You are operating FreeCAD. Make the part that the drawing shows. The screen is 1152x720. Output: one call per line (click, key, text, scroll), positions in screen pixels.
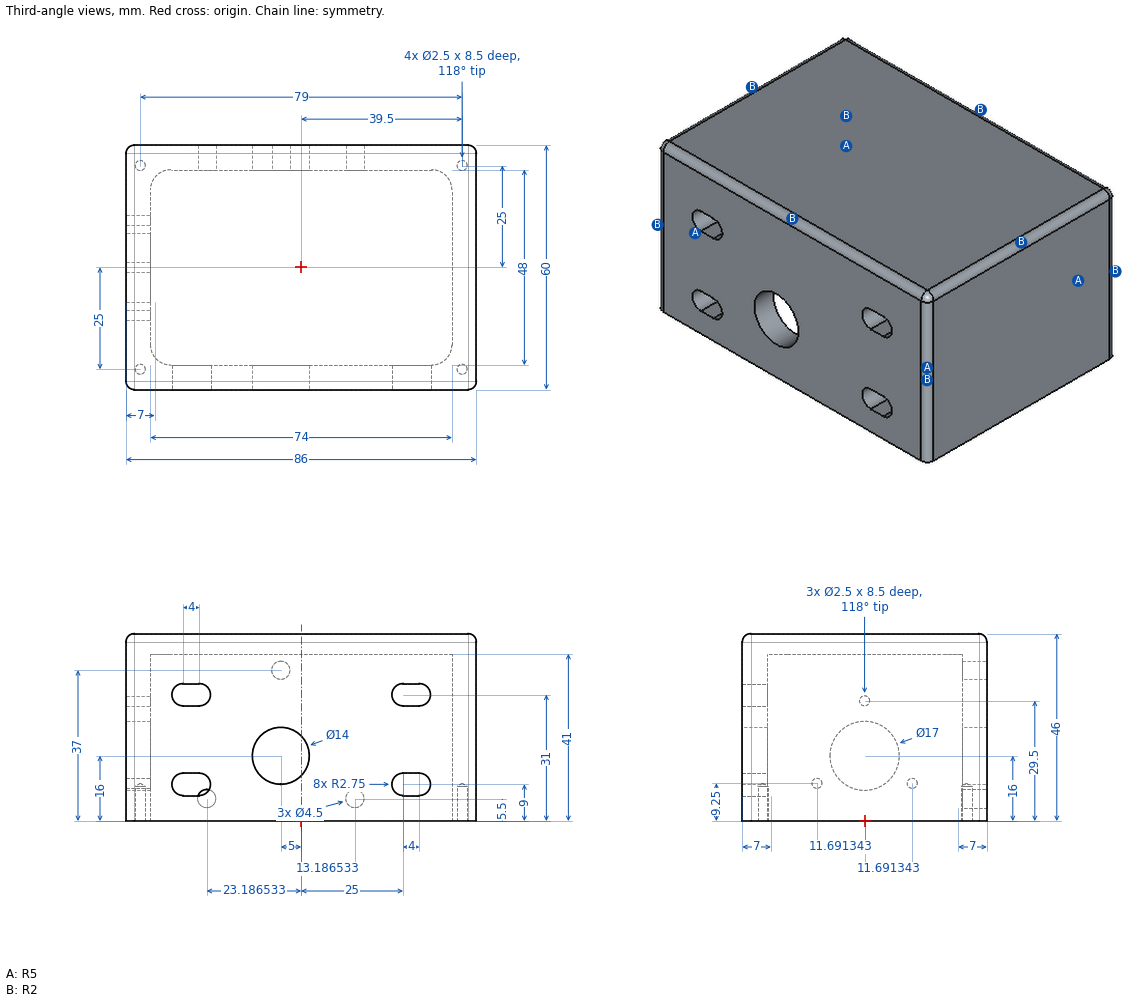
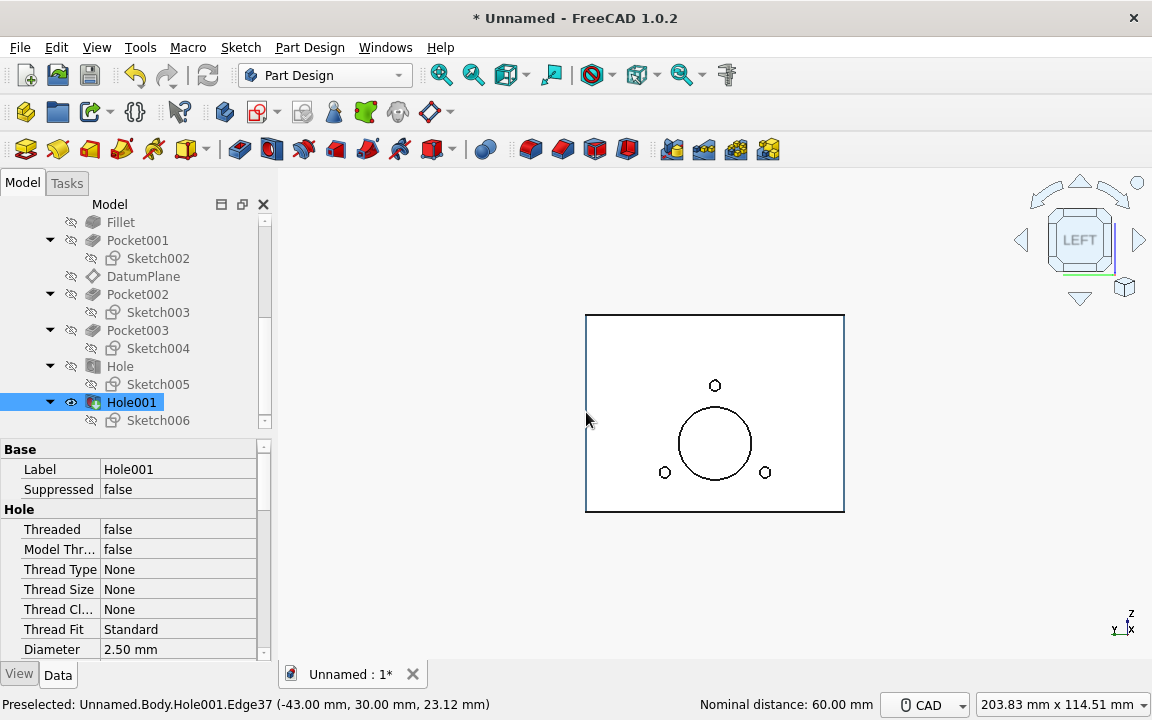
key(0)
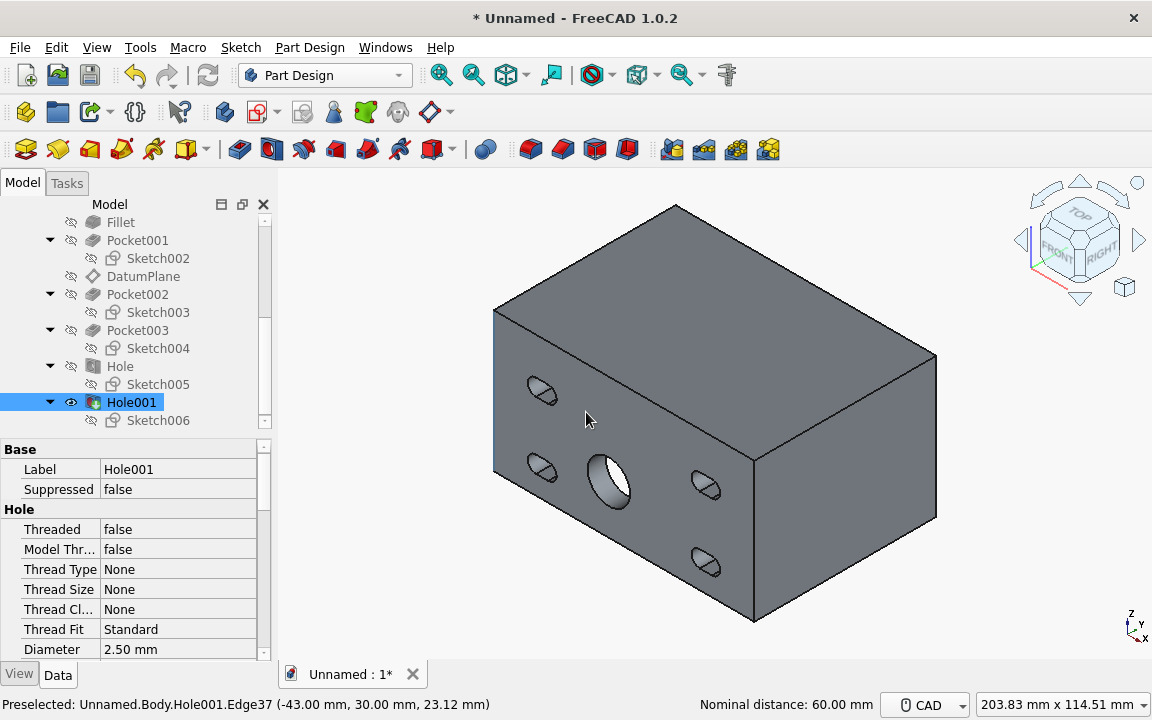
click(752, 353, ctrl)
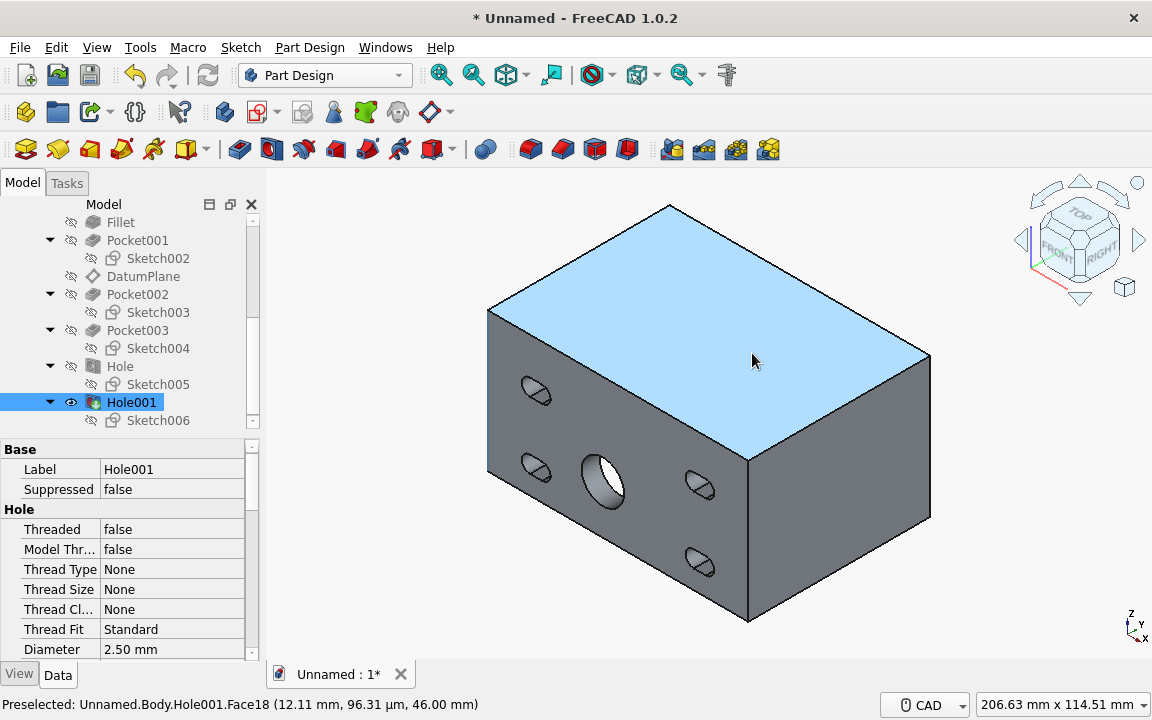
click(748, 540, ctrl)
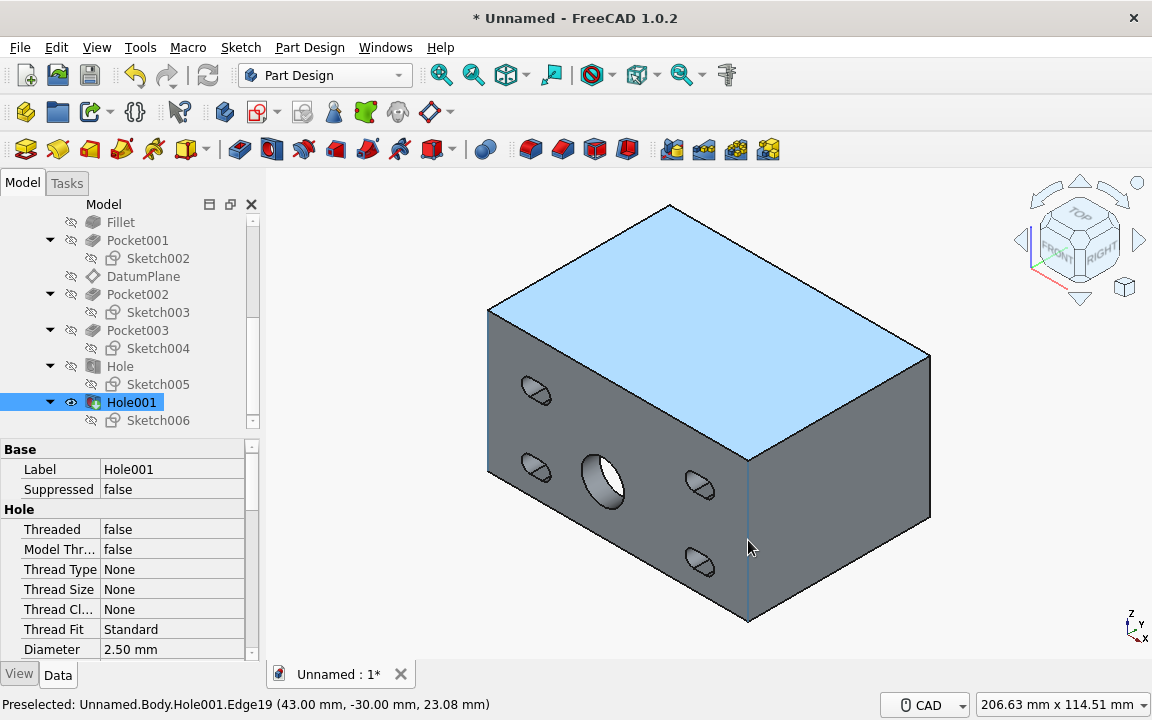
key(2)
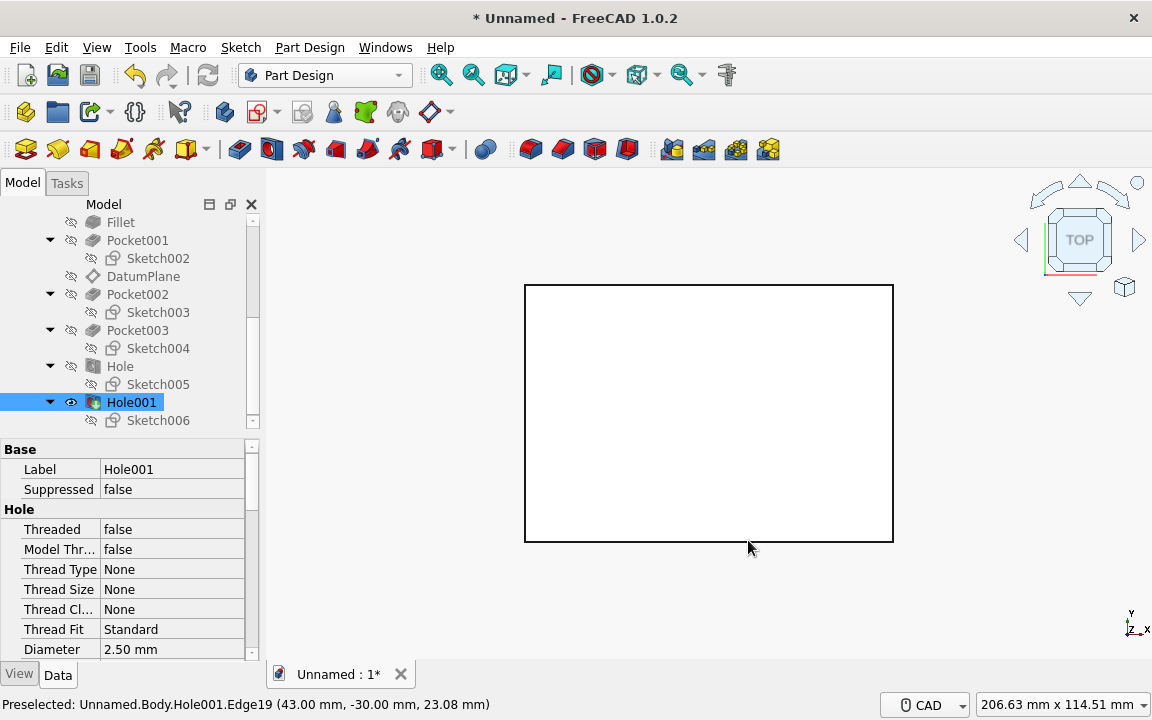
key(1)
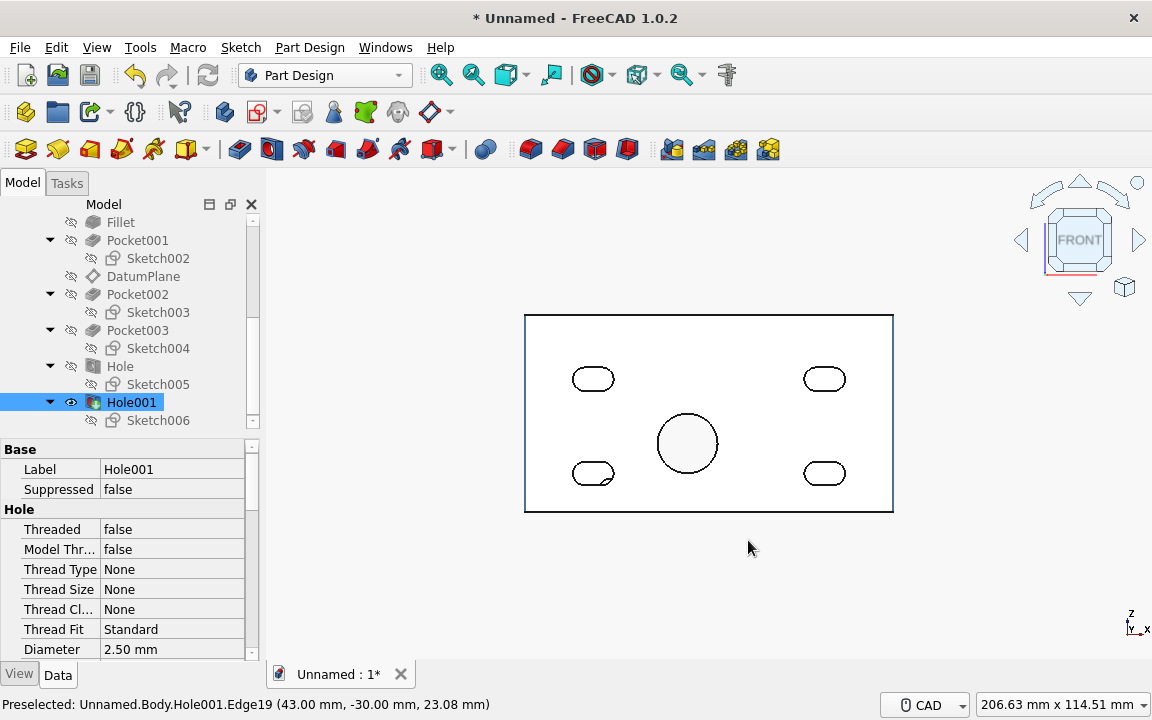
key(v)
key(f)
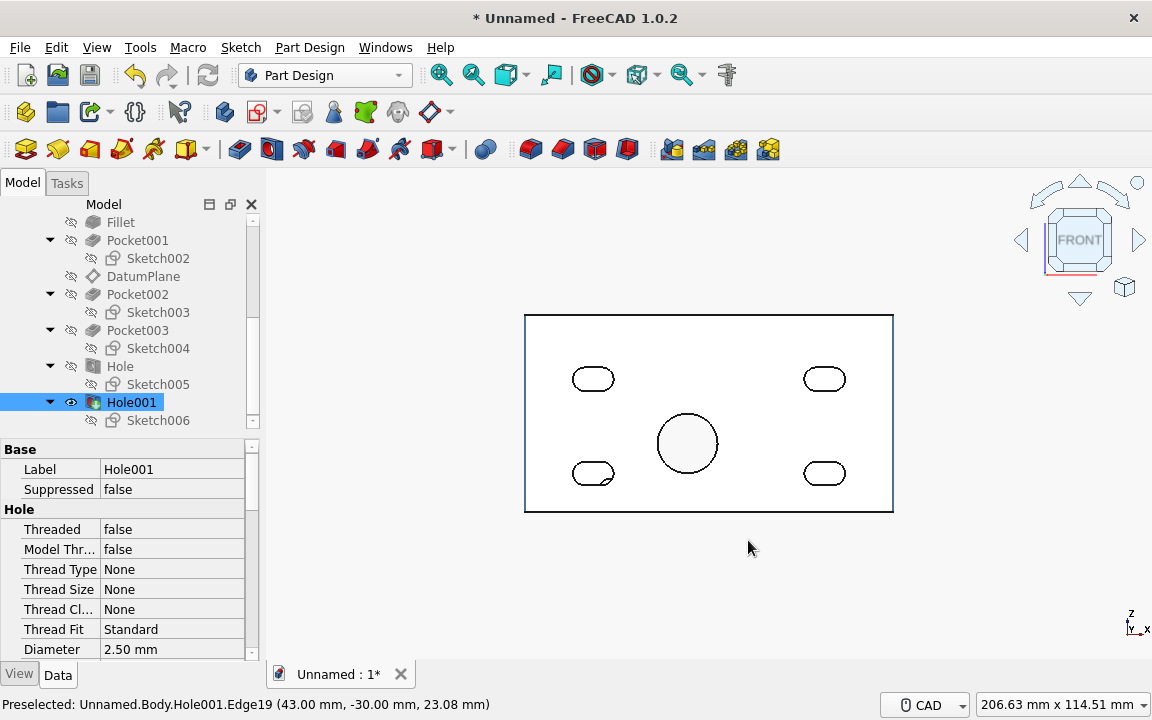
key(3)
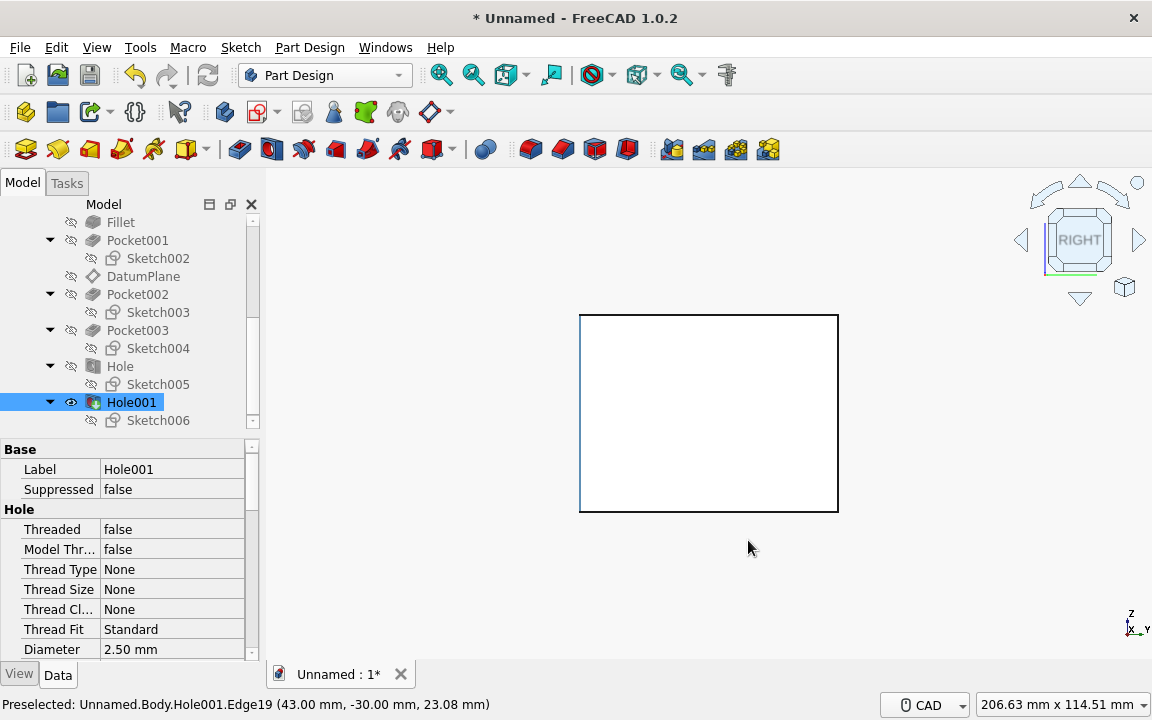
key(v)
key(f)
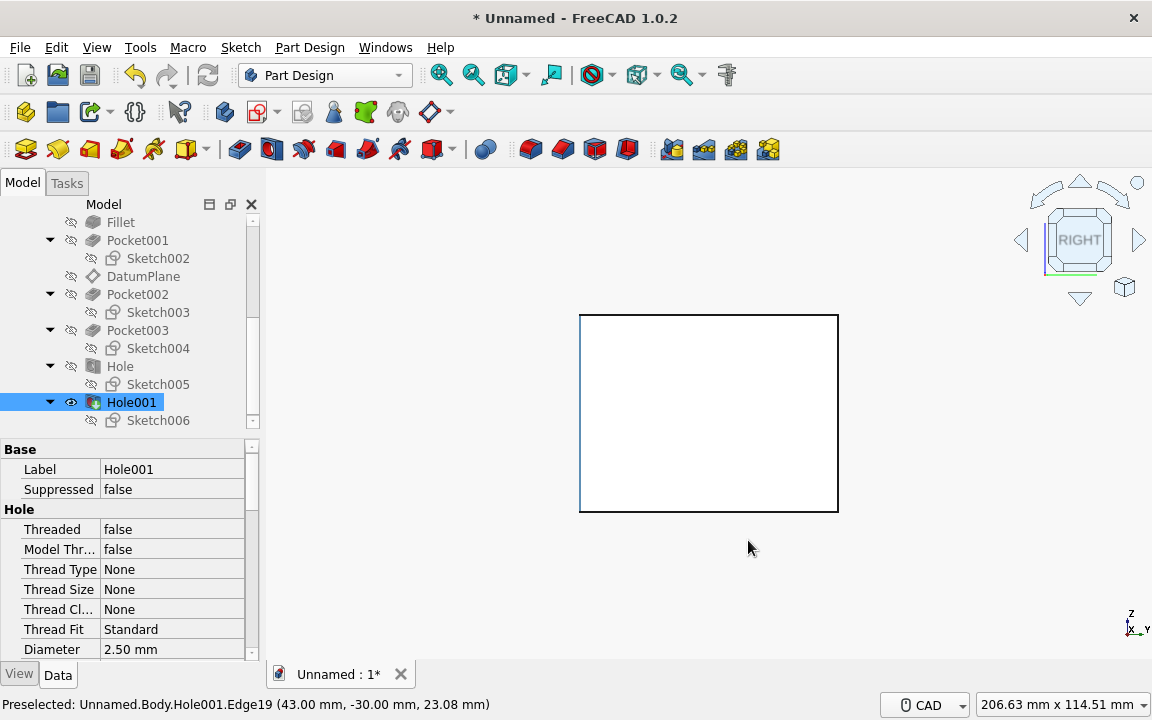
click(838, 412, ctrl)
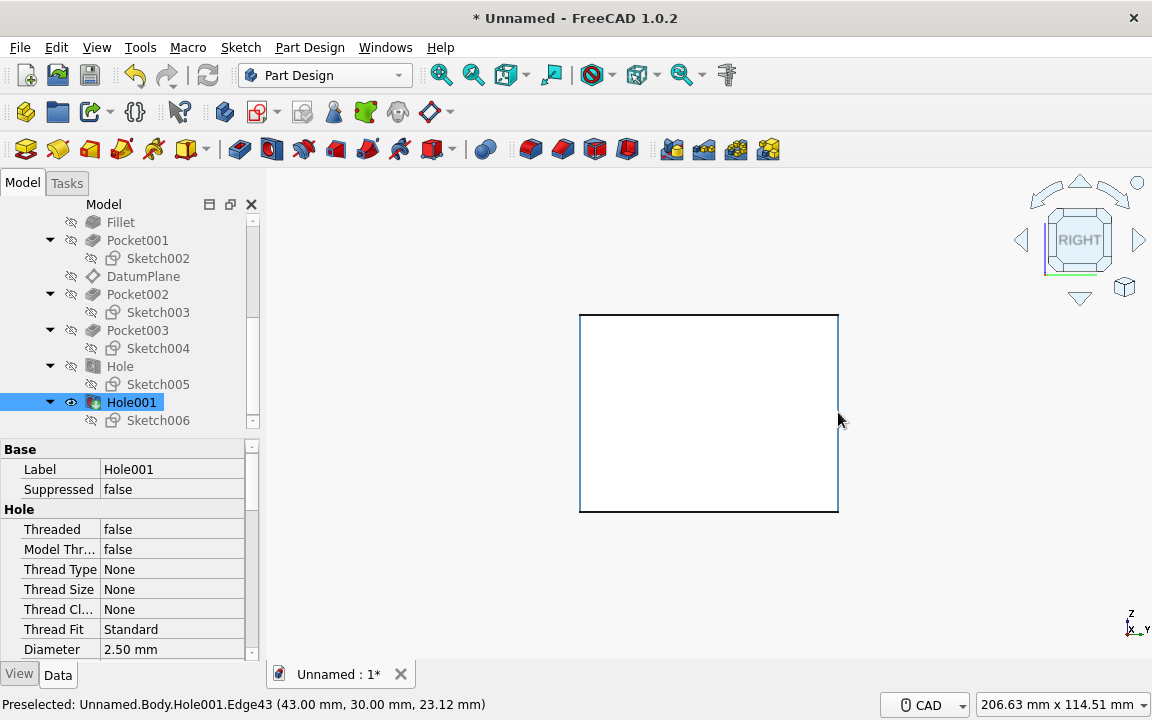
click(532, 150)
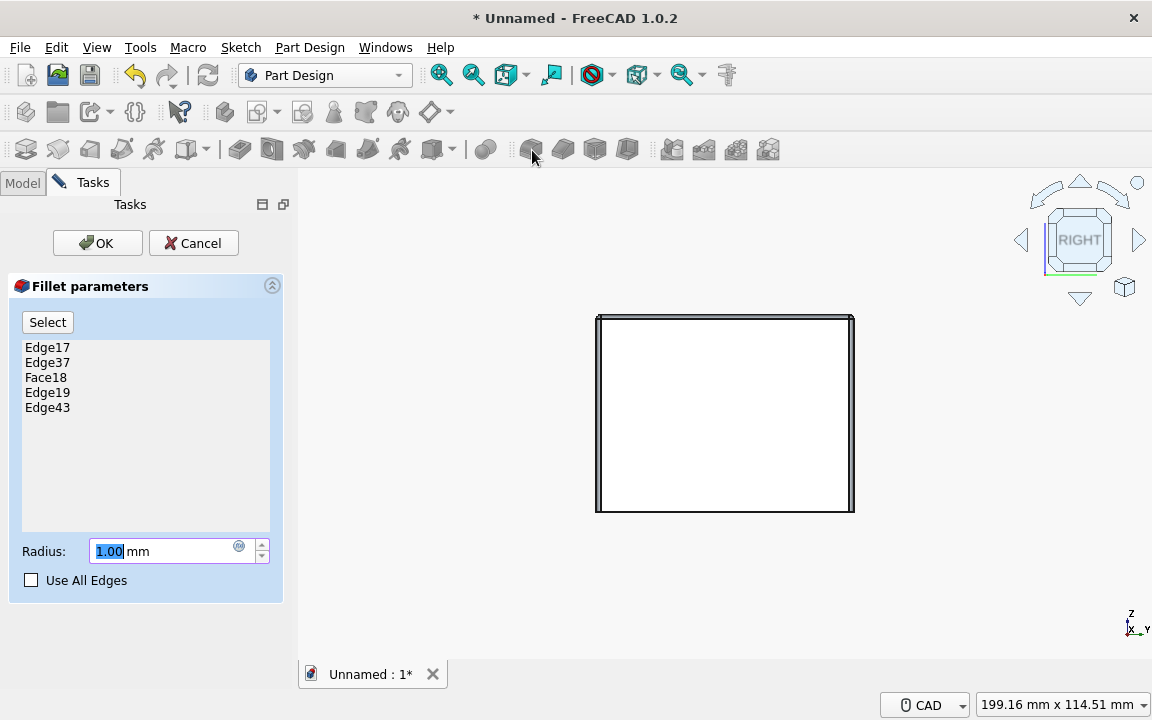
text(2)
key(Tab)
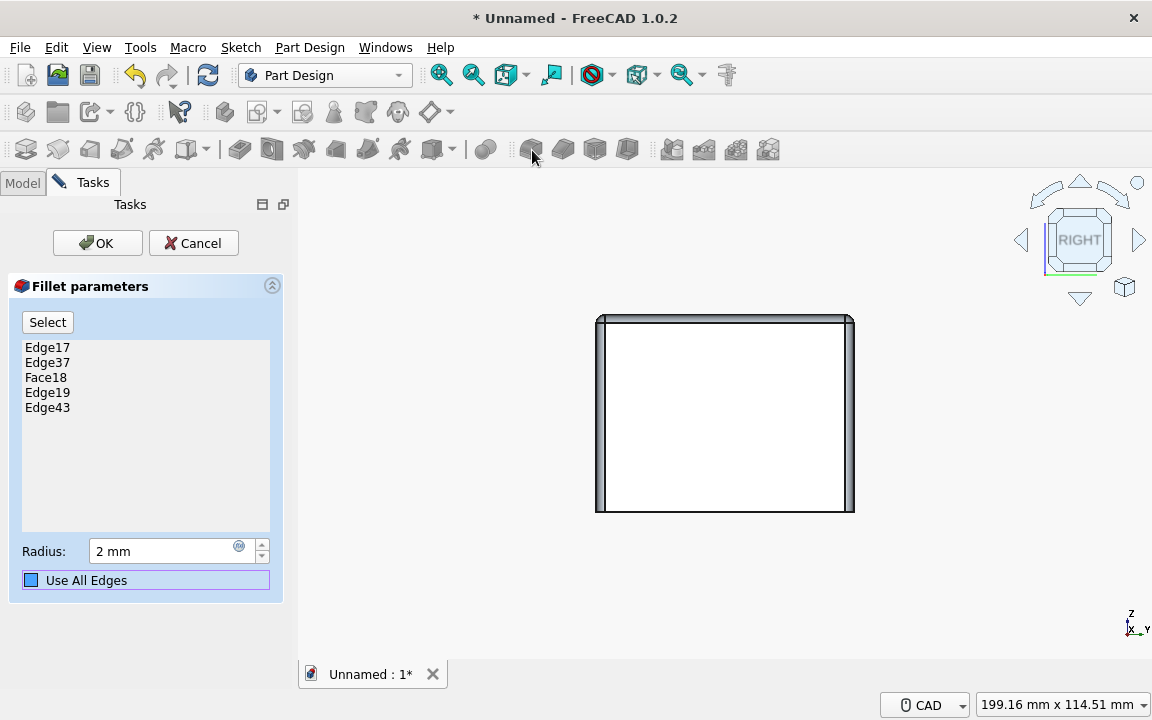
click(98, 243)